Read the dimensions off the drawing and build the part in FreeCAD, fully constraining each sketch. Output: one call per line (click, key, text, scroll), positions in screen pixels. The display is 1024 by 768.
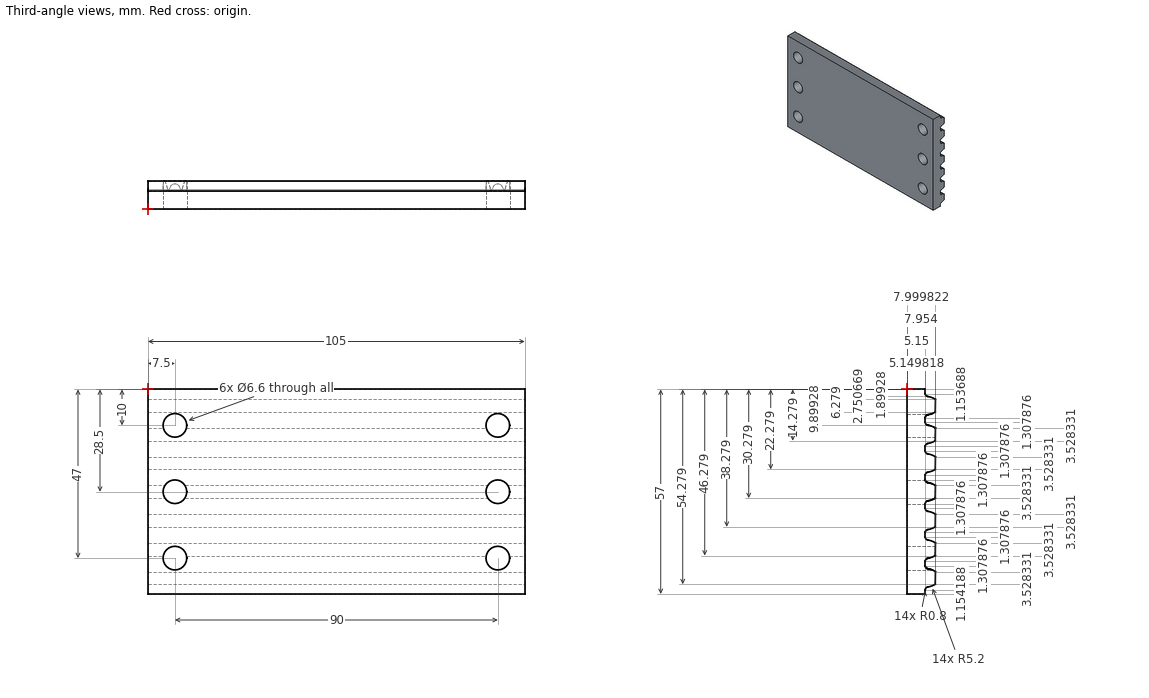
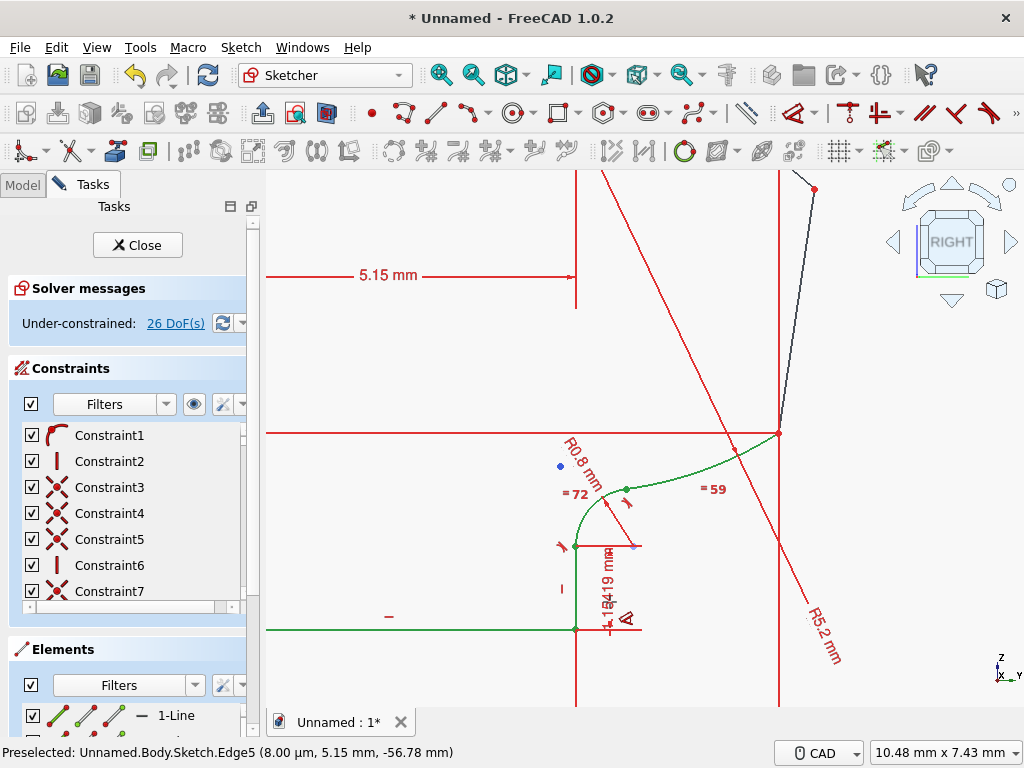
scroll(585, 625, down, 12)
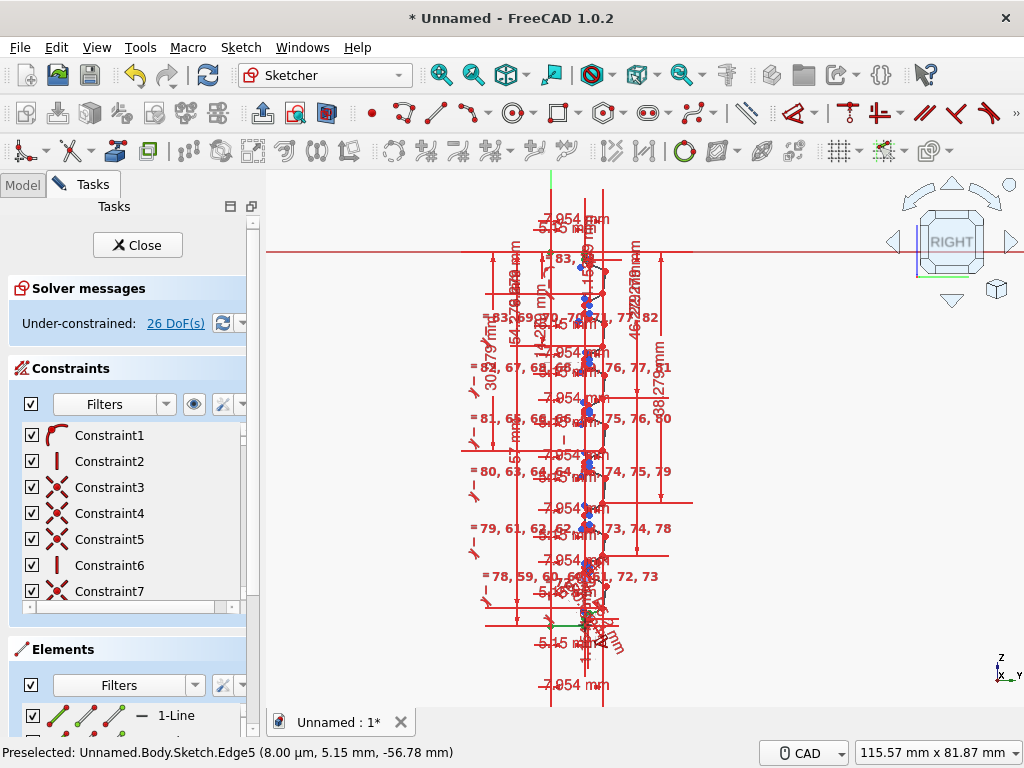
scroll(585, 571, up, 12)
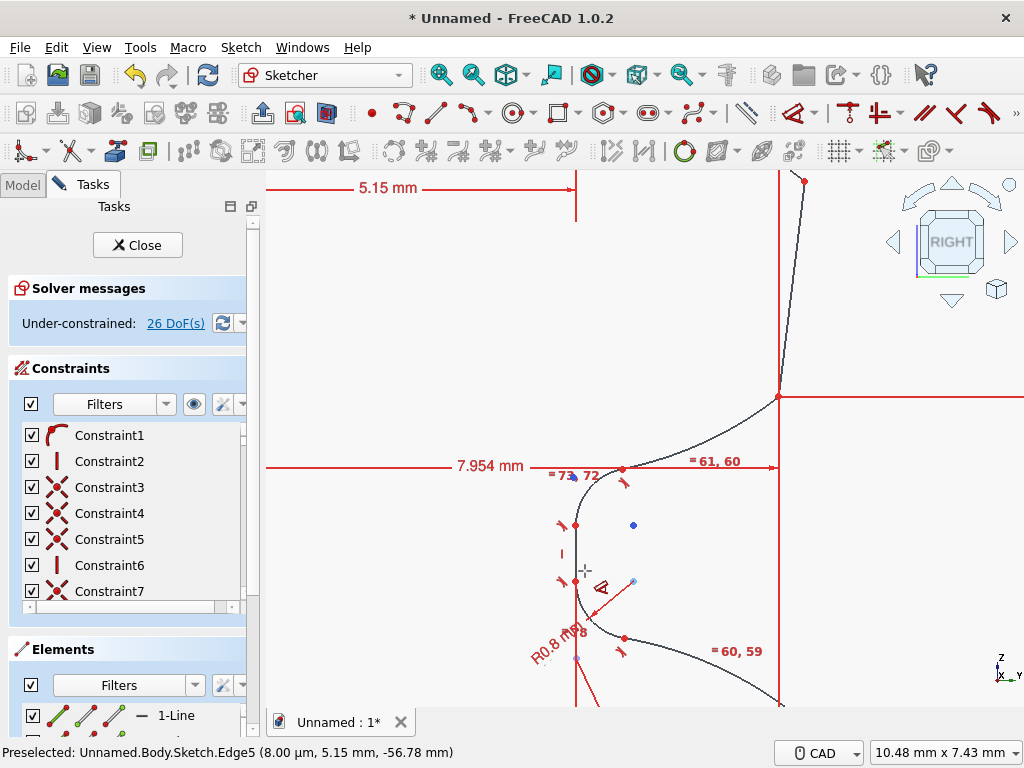
click(576, 565)
click(610, 553)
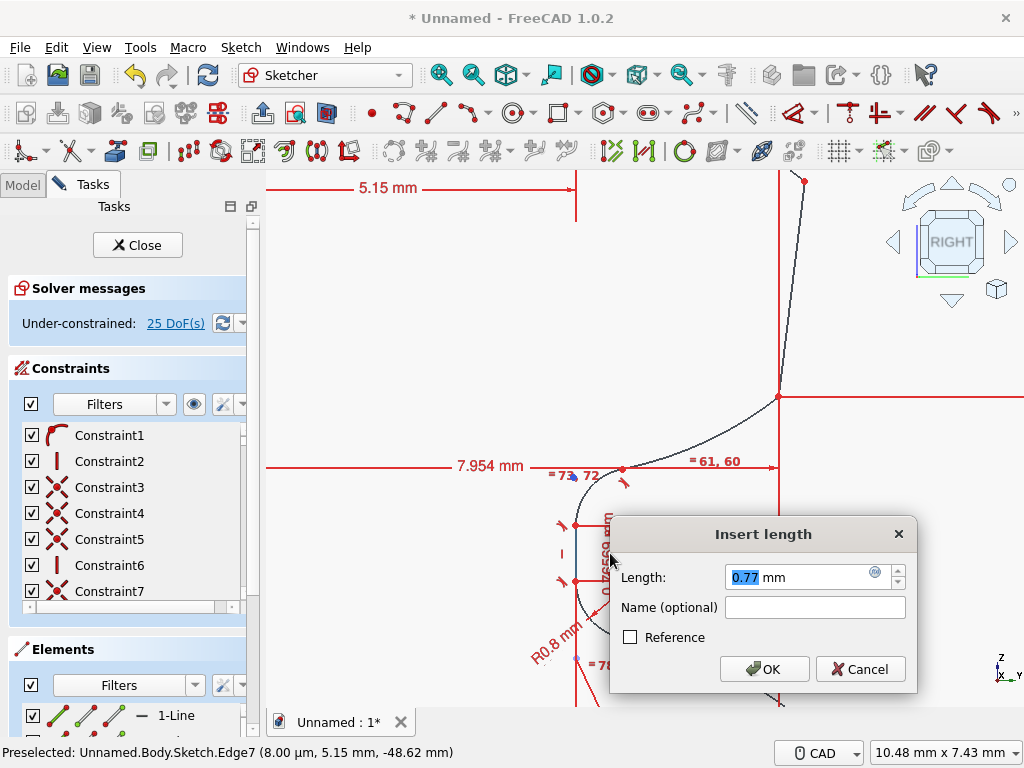
text(1.307876)
key(Return)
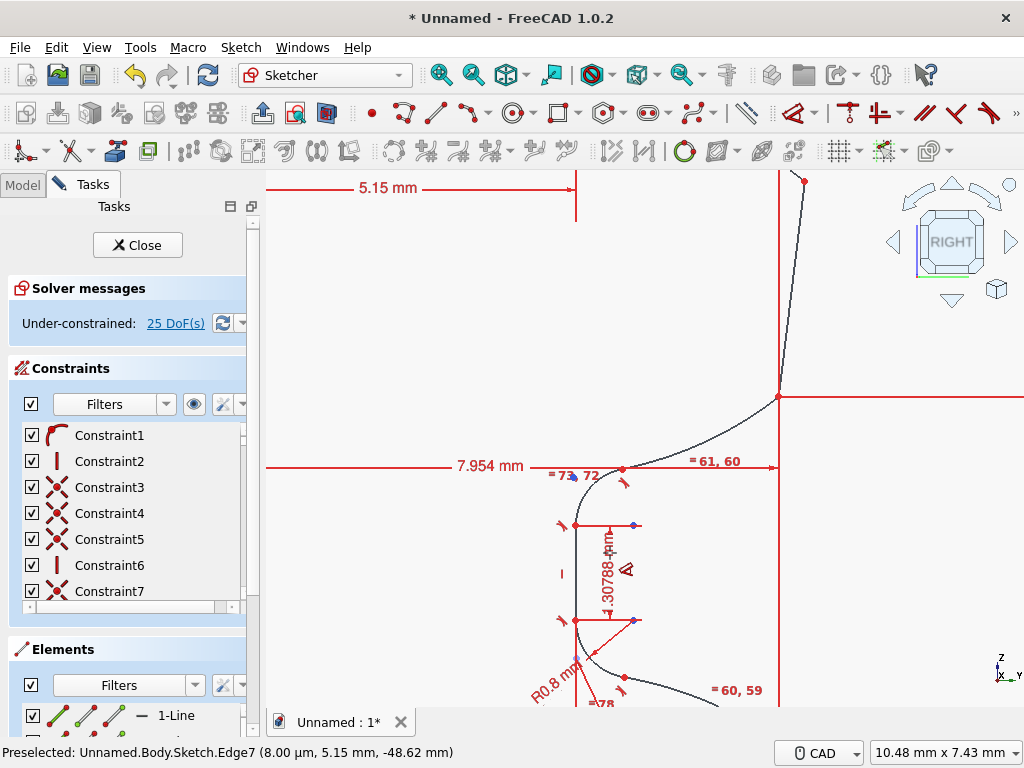
scroll(585, 571, down, 12)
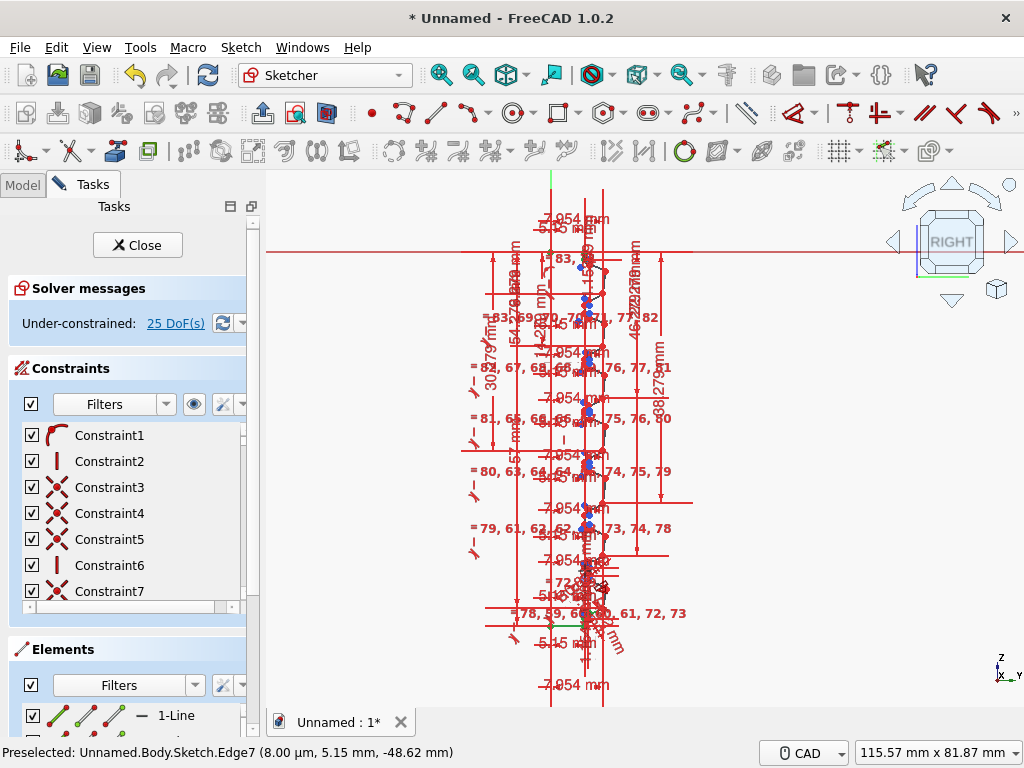
scroll(585, 522, up, 9)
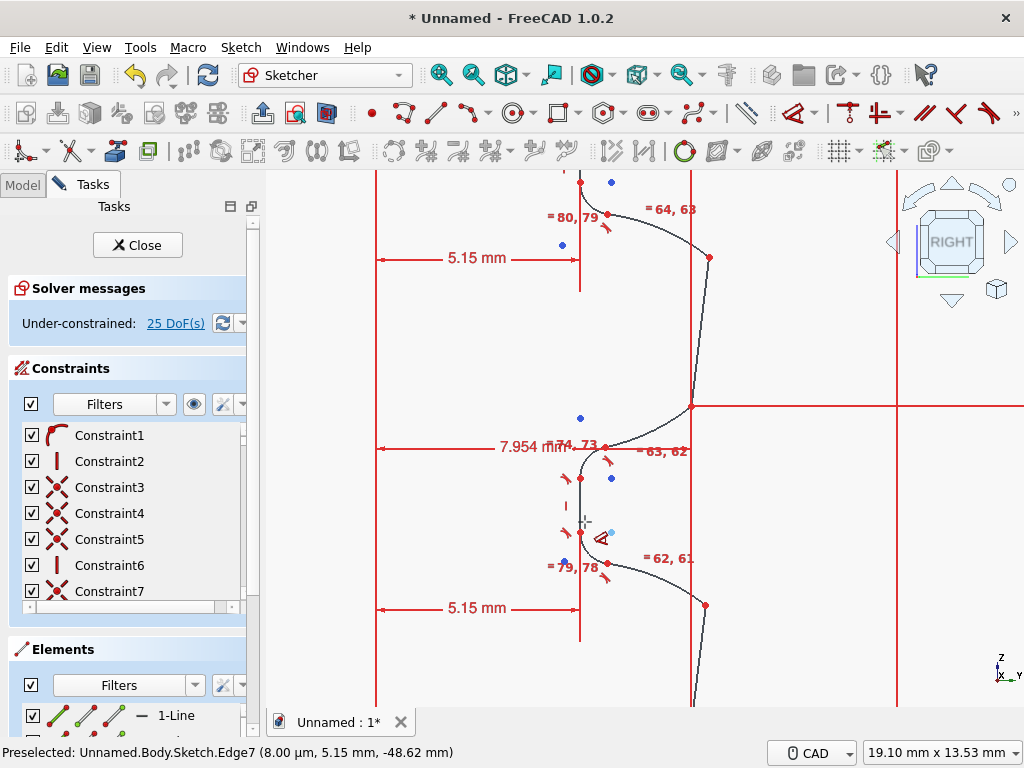
click(580, 516)
click(614, 505)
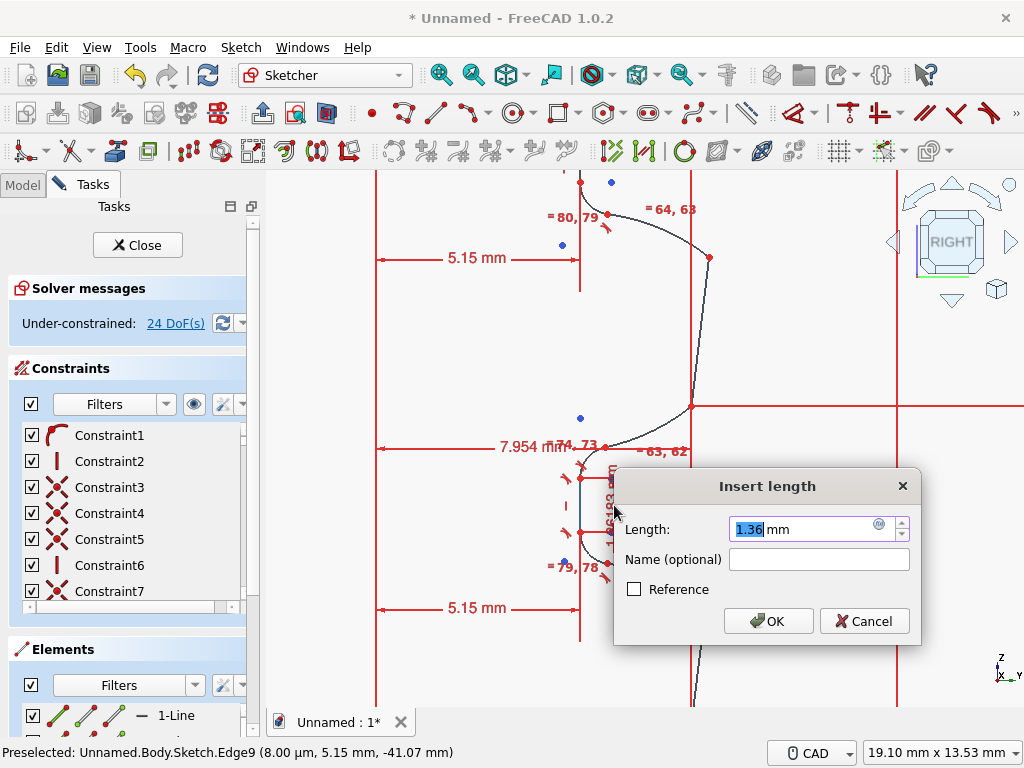
text(1.307876)
key(Return)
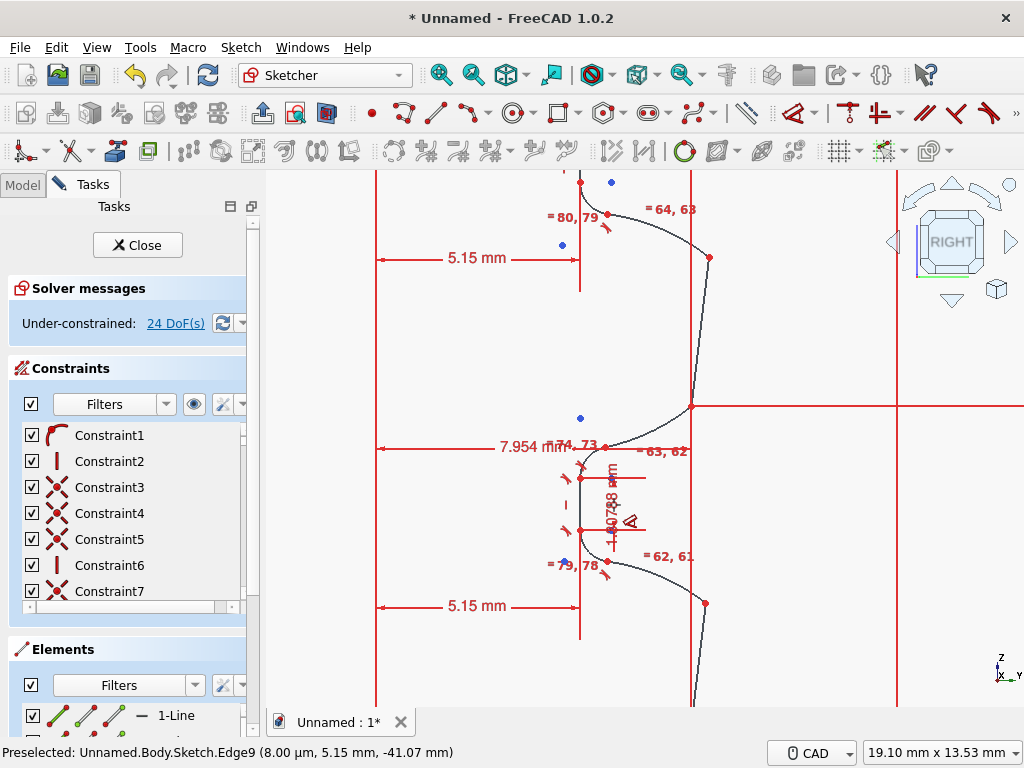
scroll(585, 522, down, 9)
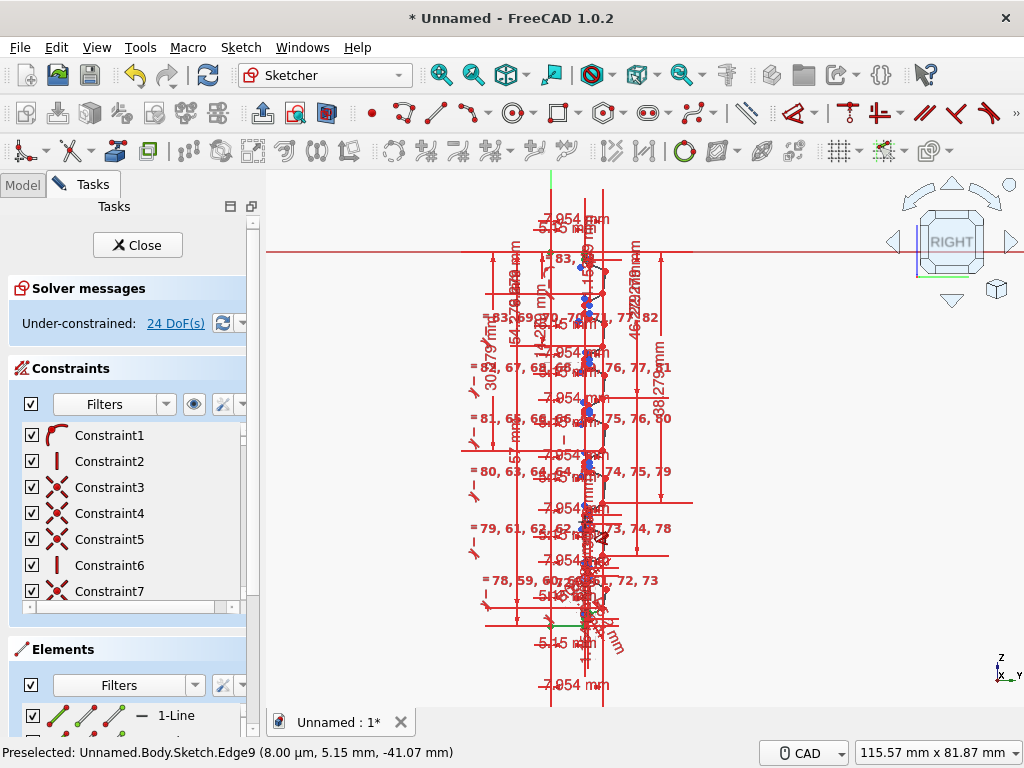
scroll(585, 465, up, 11)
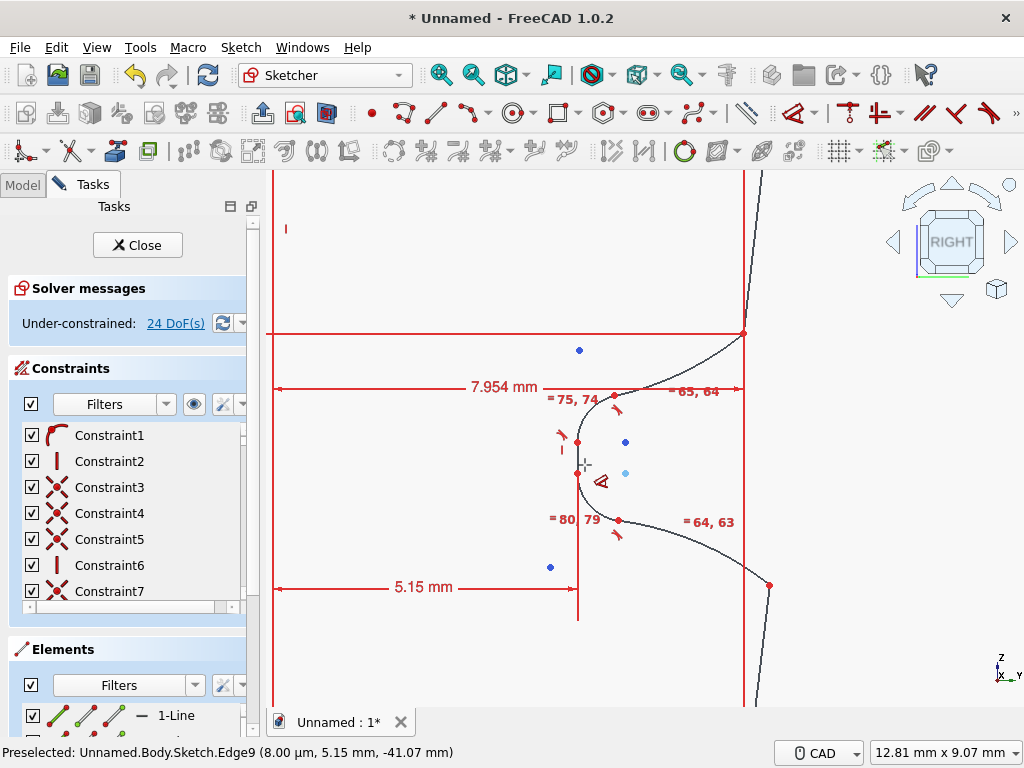
click(578, 458)
click(612, 458)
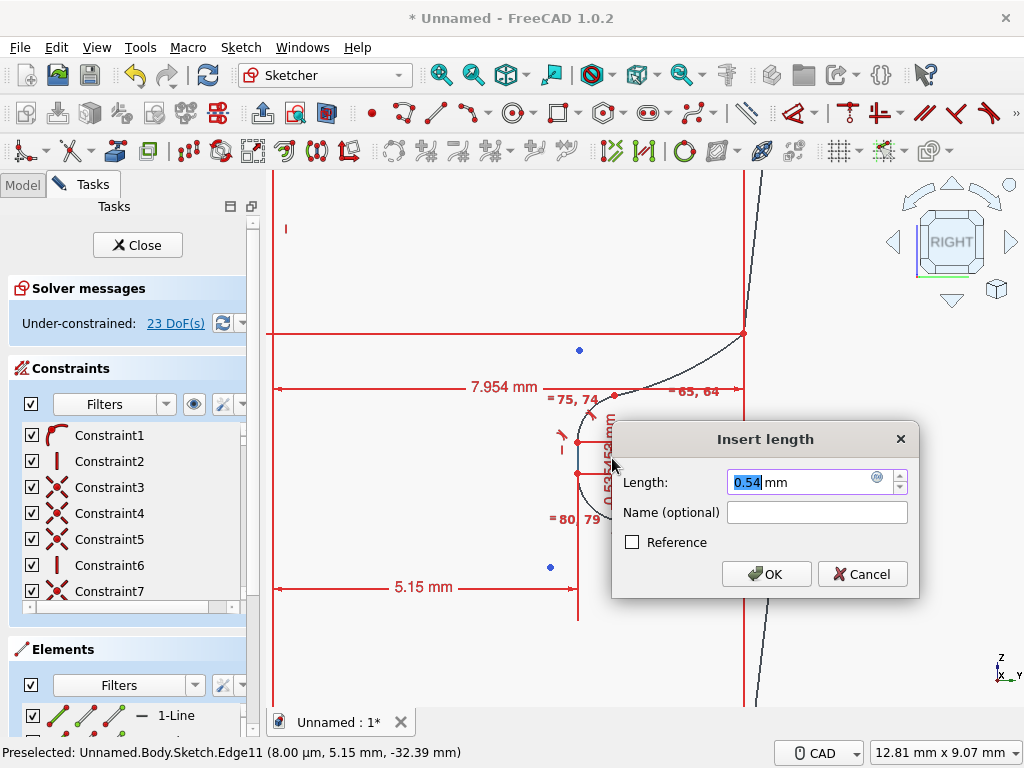
text(1.307876)
key(Return)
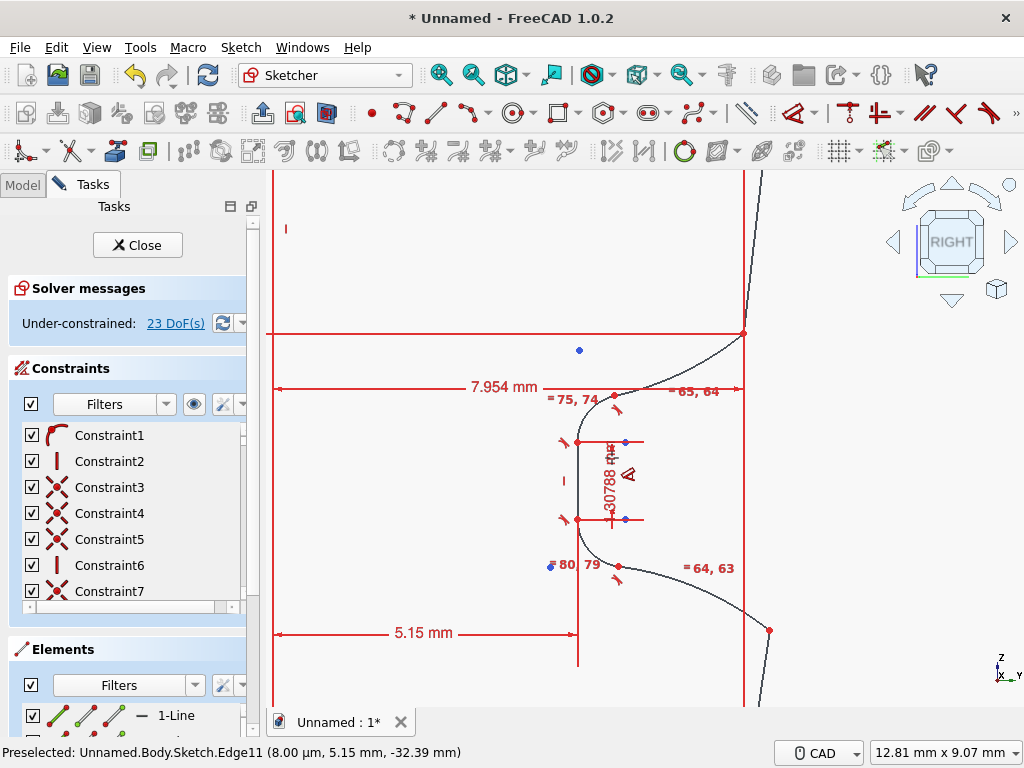
scroll(585, 465, down, 11)